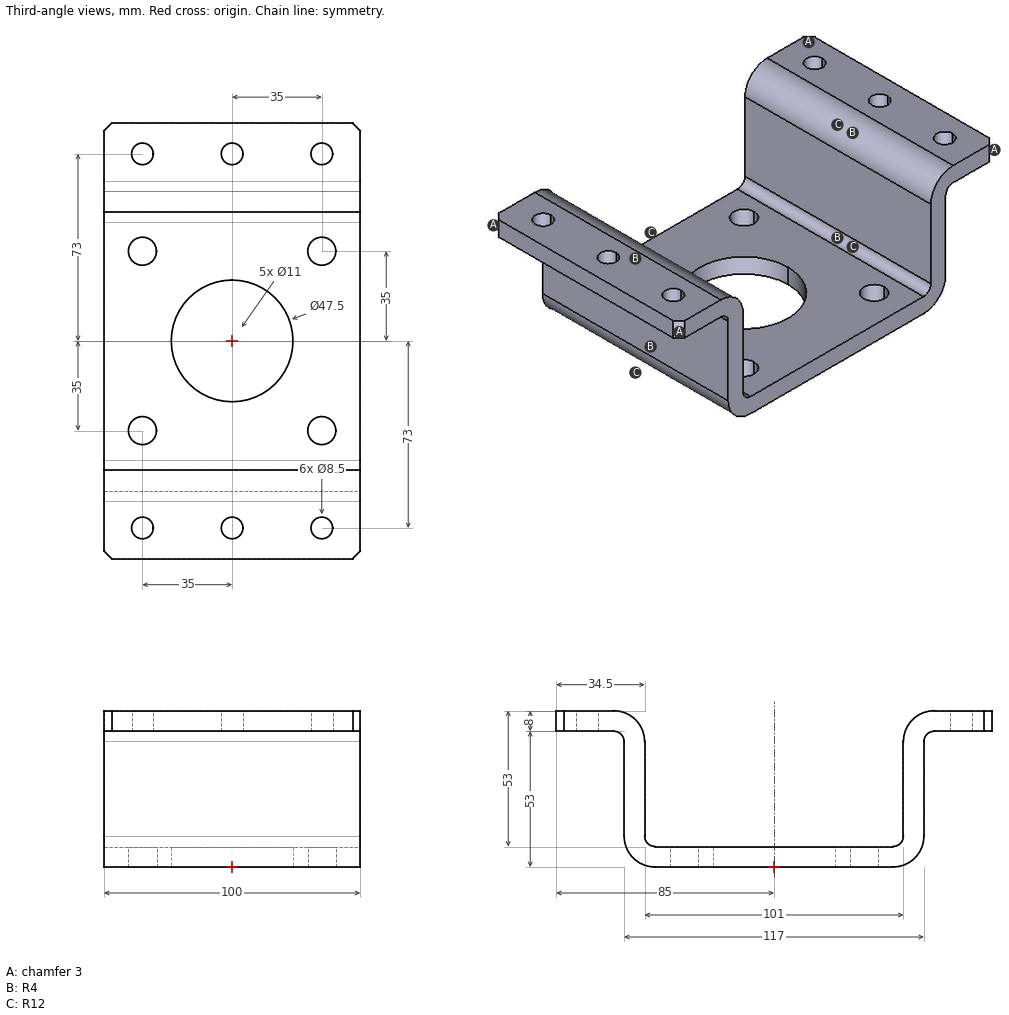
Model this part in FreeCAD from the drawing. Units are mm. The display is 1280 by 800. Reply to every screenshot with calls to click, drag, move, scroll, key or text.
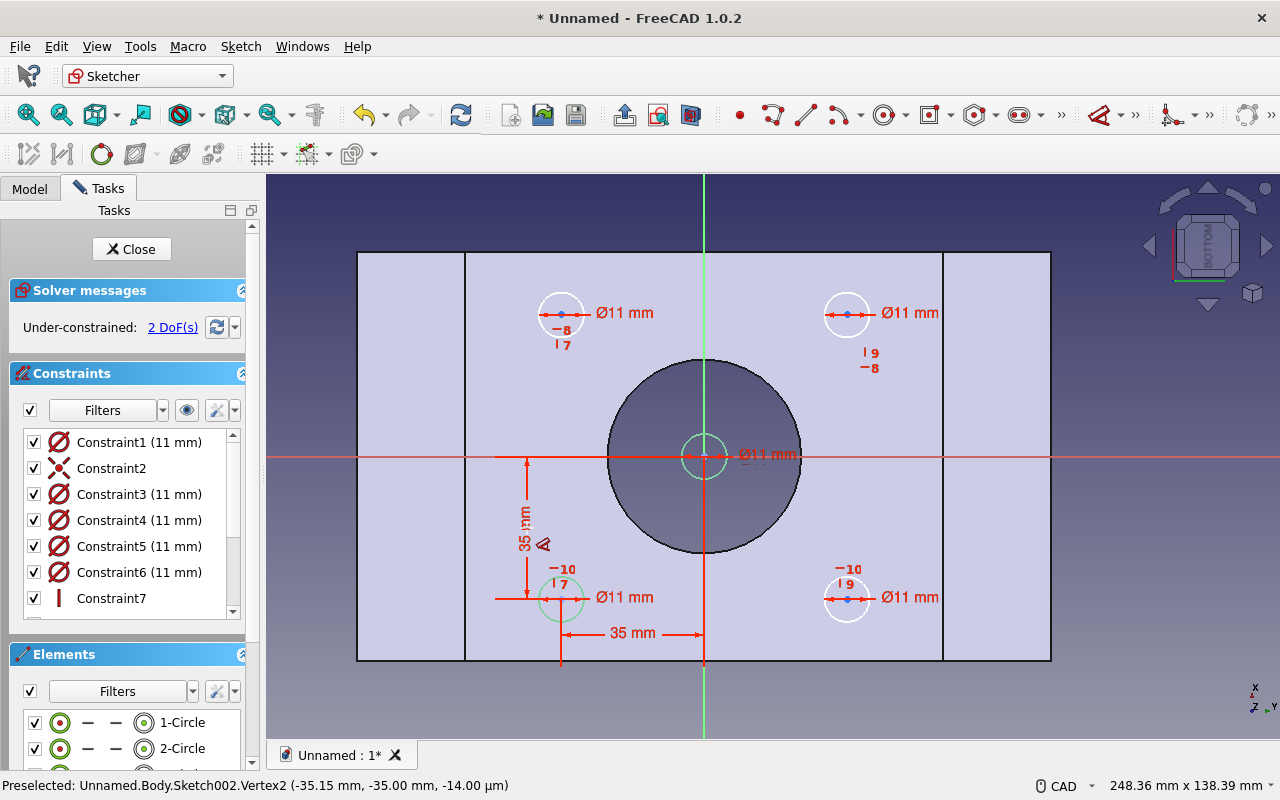
click(847, 315)
click(776, 281)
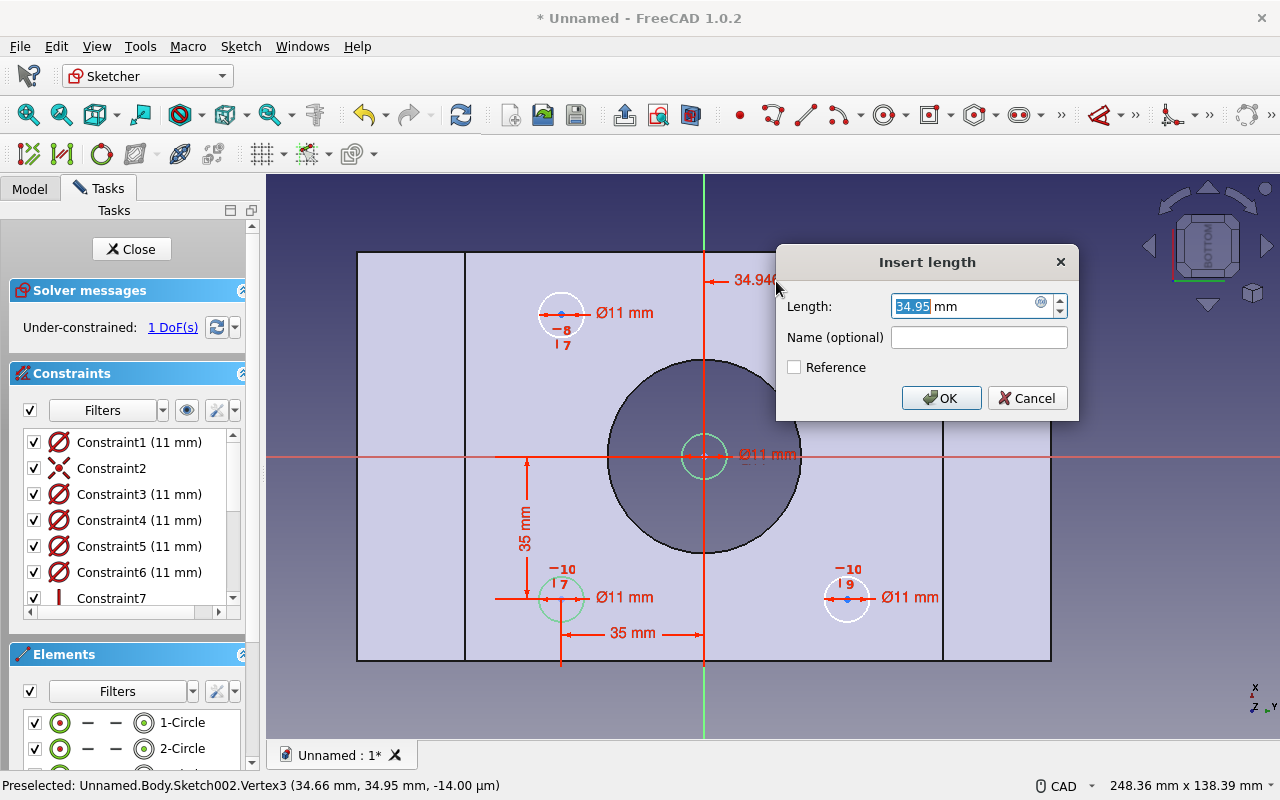
text(35)
key(Return)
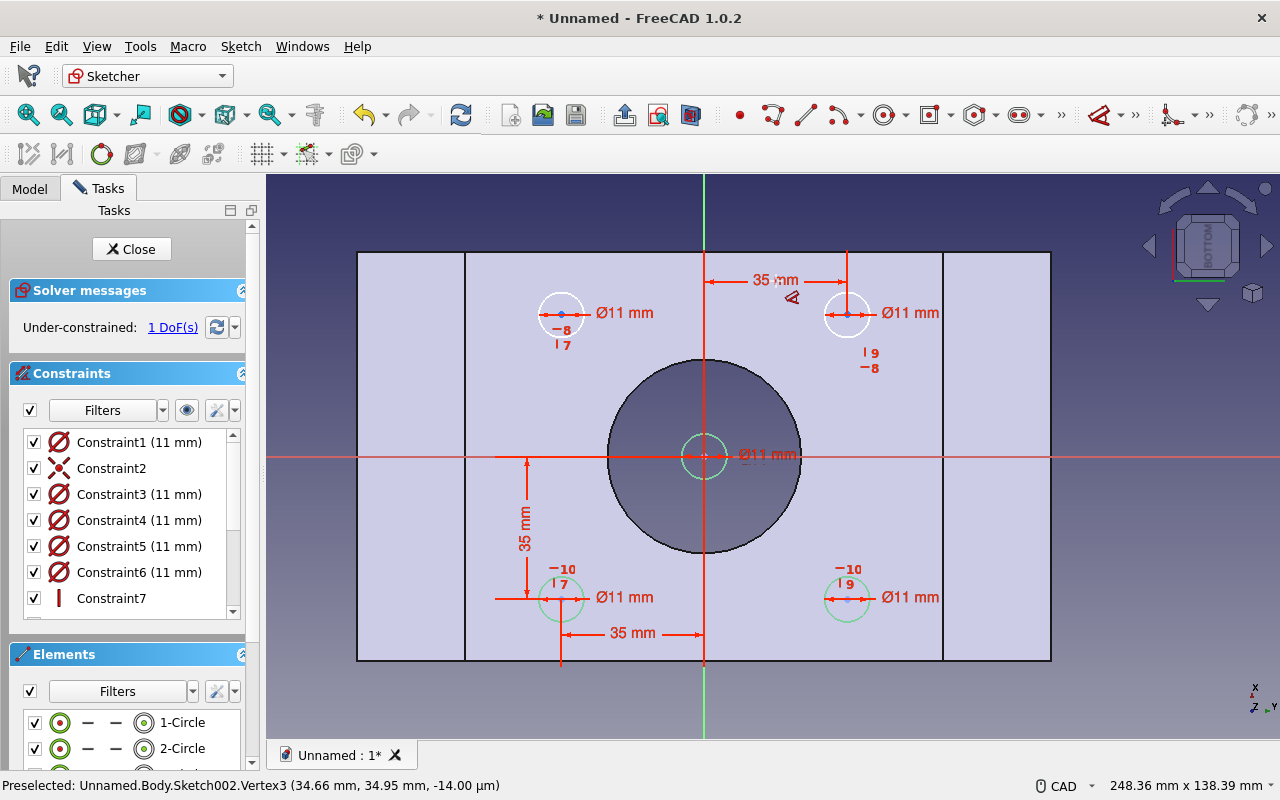
click(847, 315)
click(881, 386)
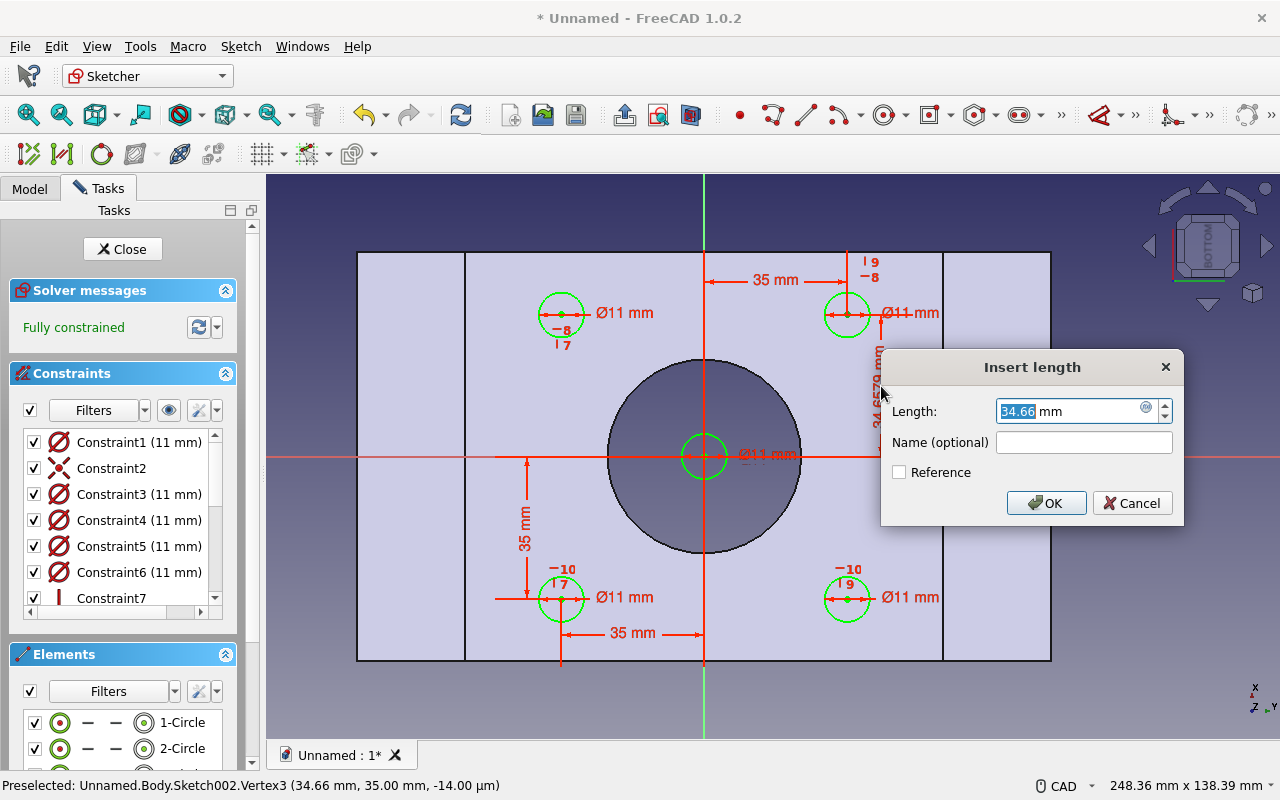
text(35)
key(Return)
key(Escape)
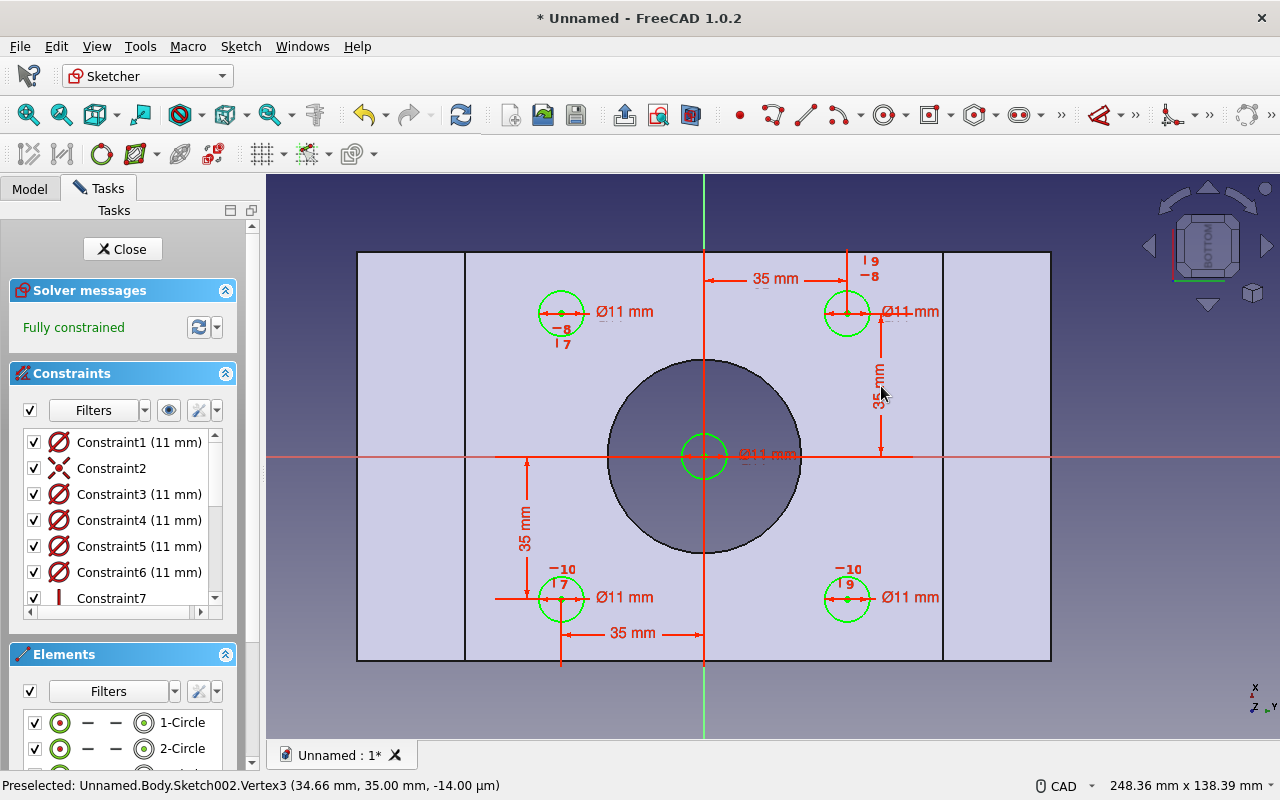
click(123, 249)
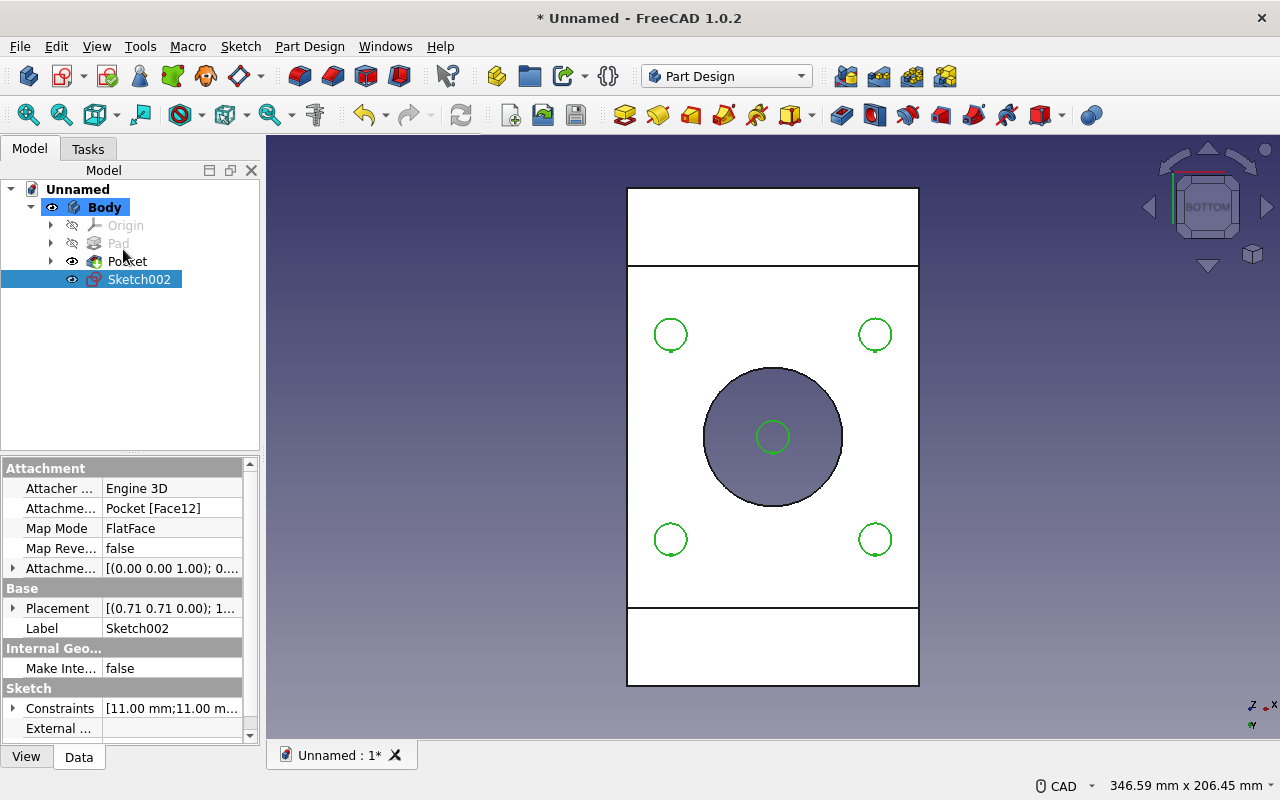
click(842, 116)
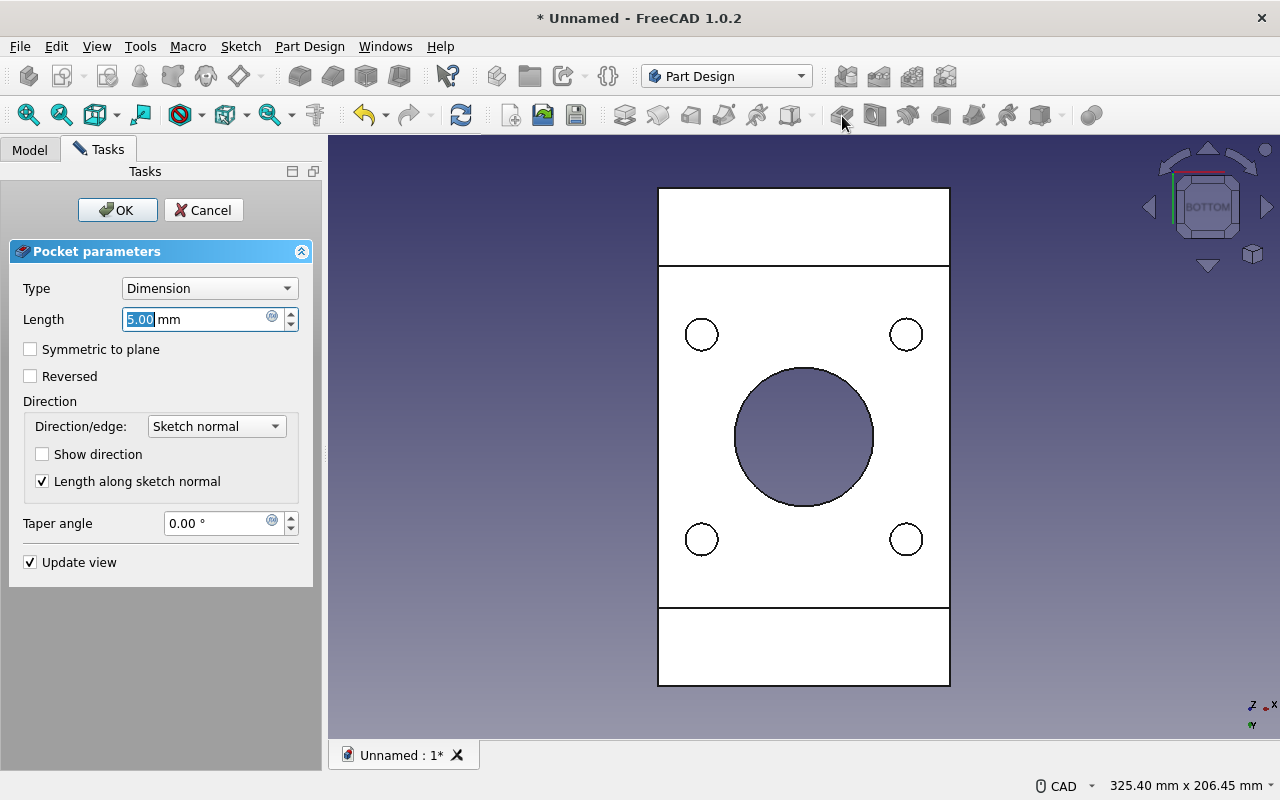
click(210, 288)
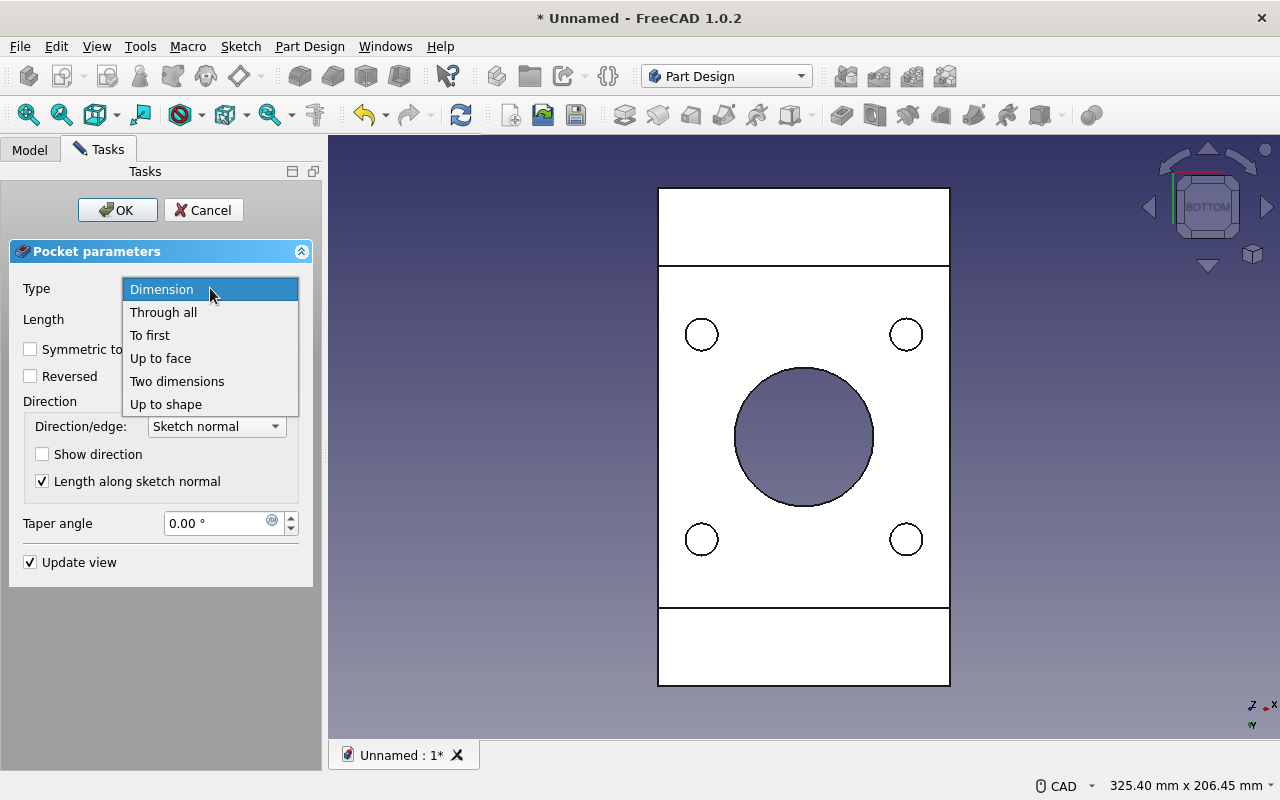
click(208, 312)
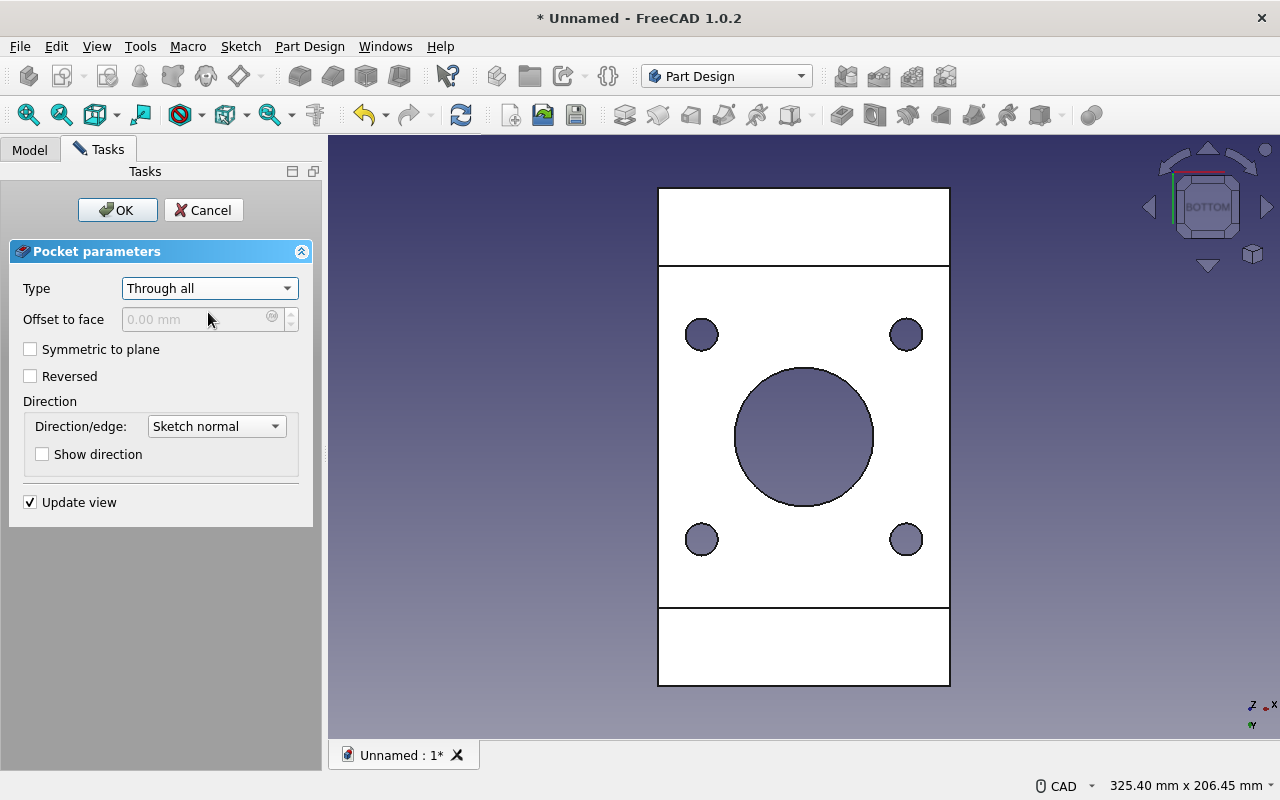
click(118, 210)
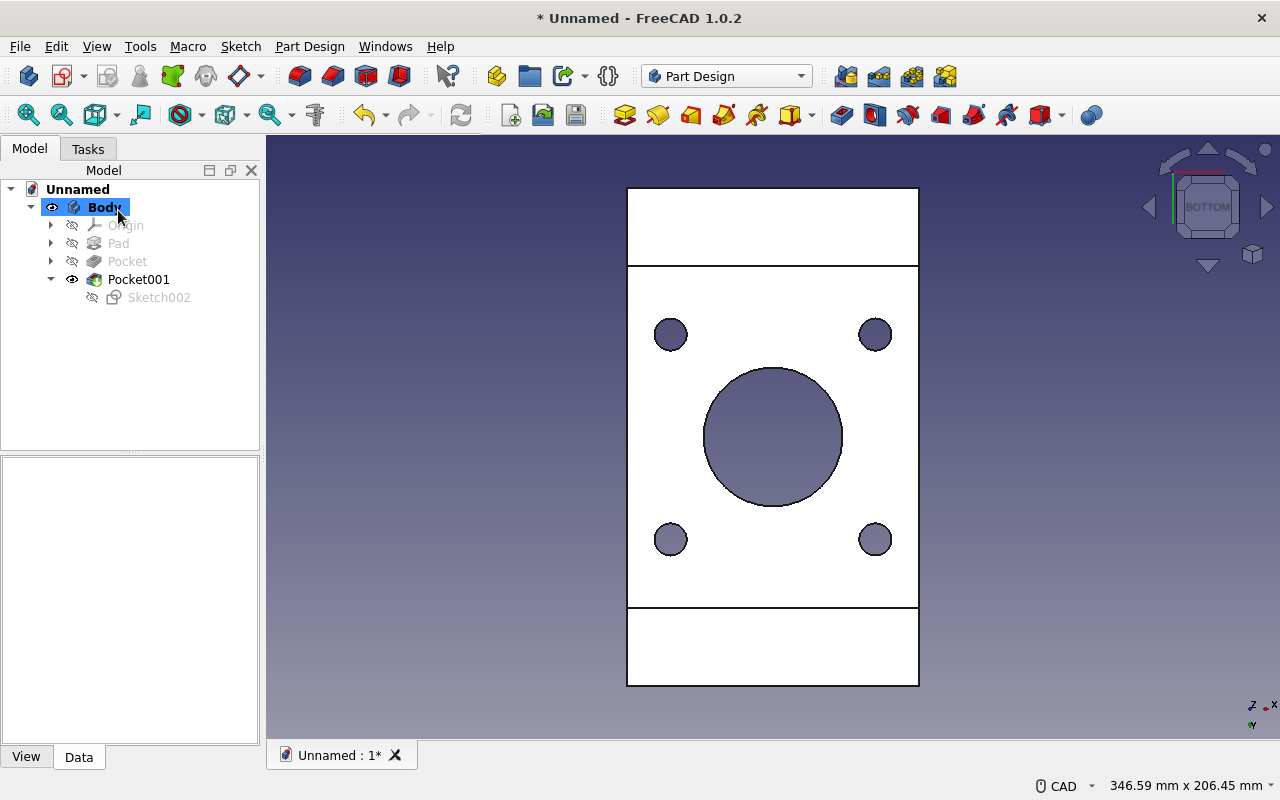
click(815, 646)